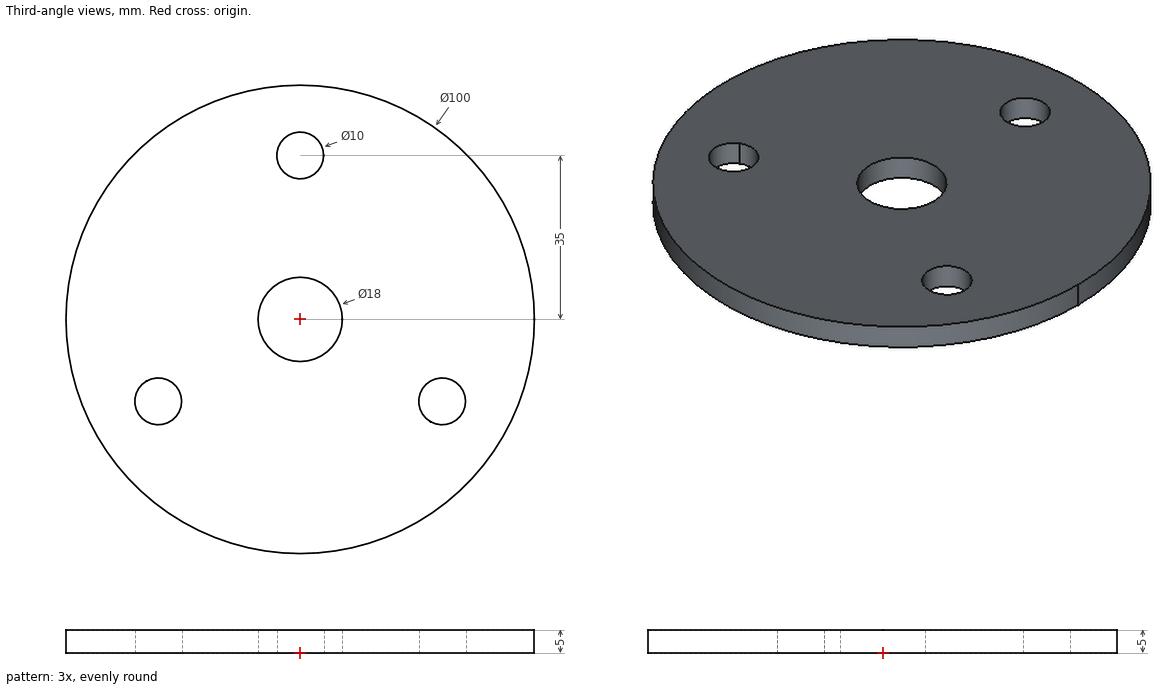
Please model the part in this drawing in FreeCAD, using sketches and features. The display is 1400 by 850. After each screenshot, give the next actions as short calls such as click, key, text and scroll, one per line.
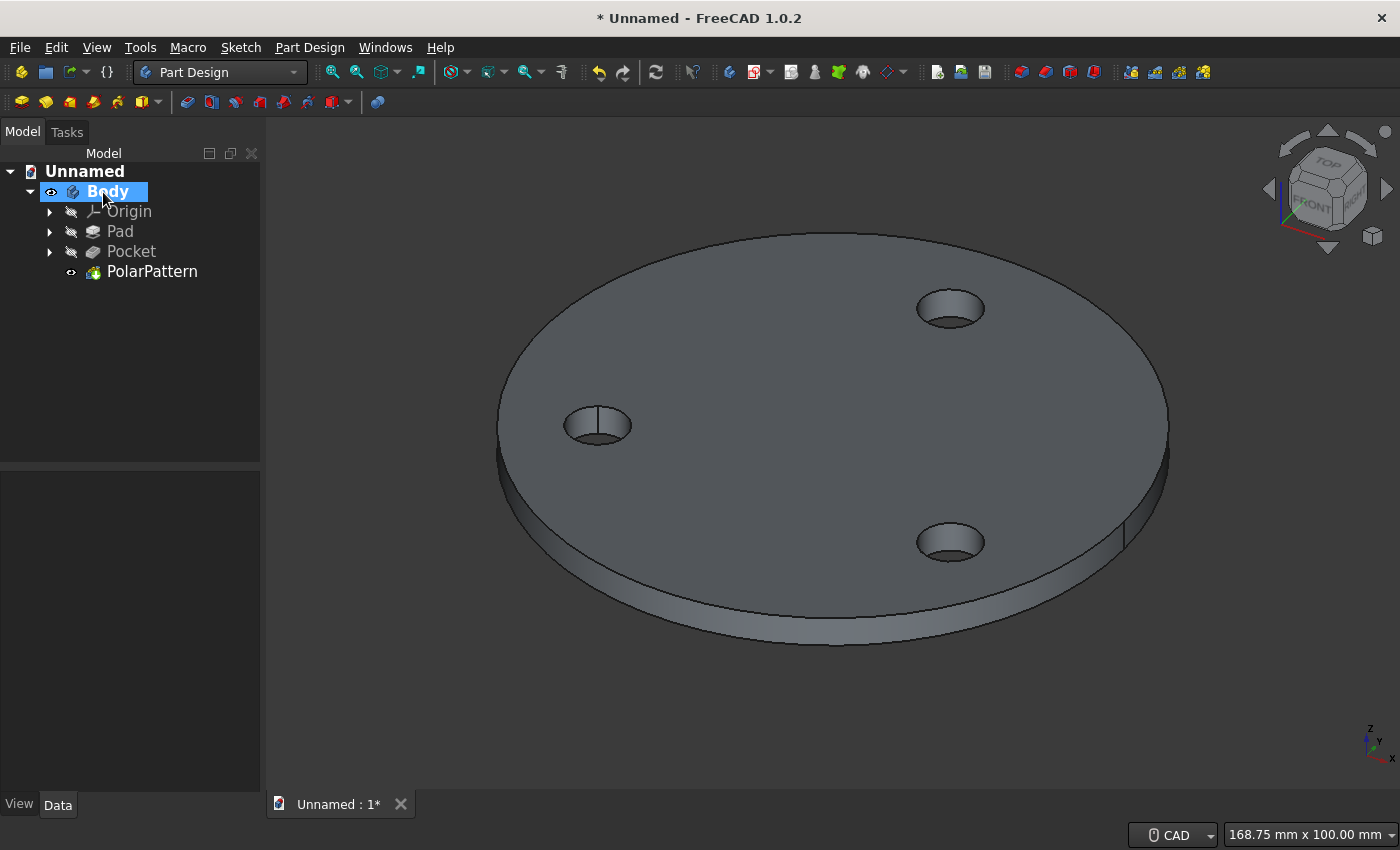
click(833, 424)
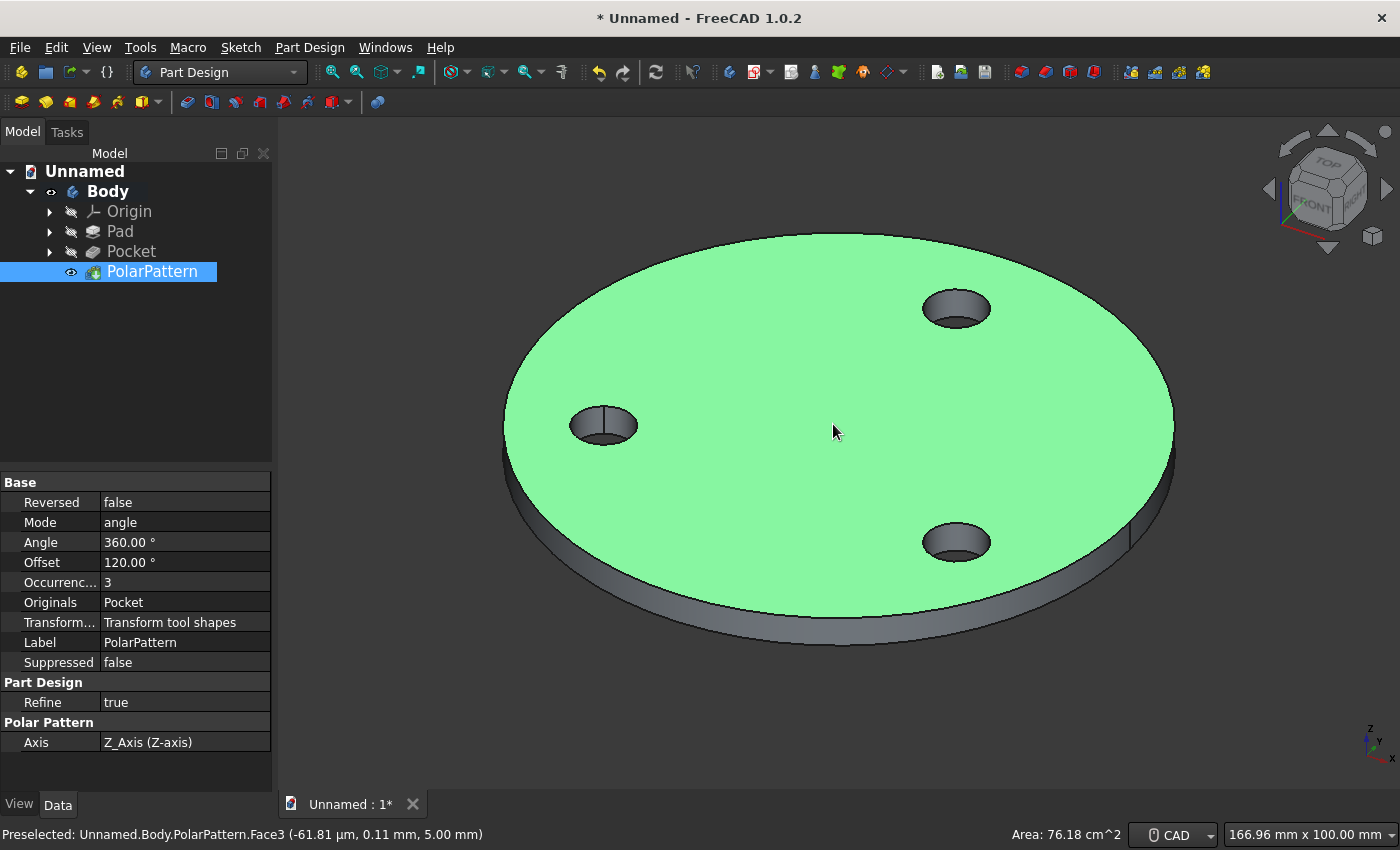
click(754, 72)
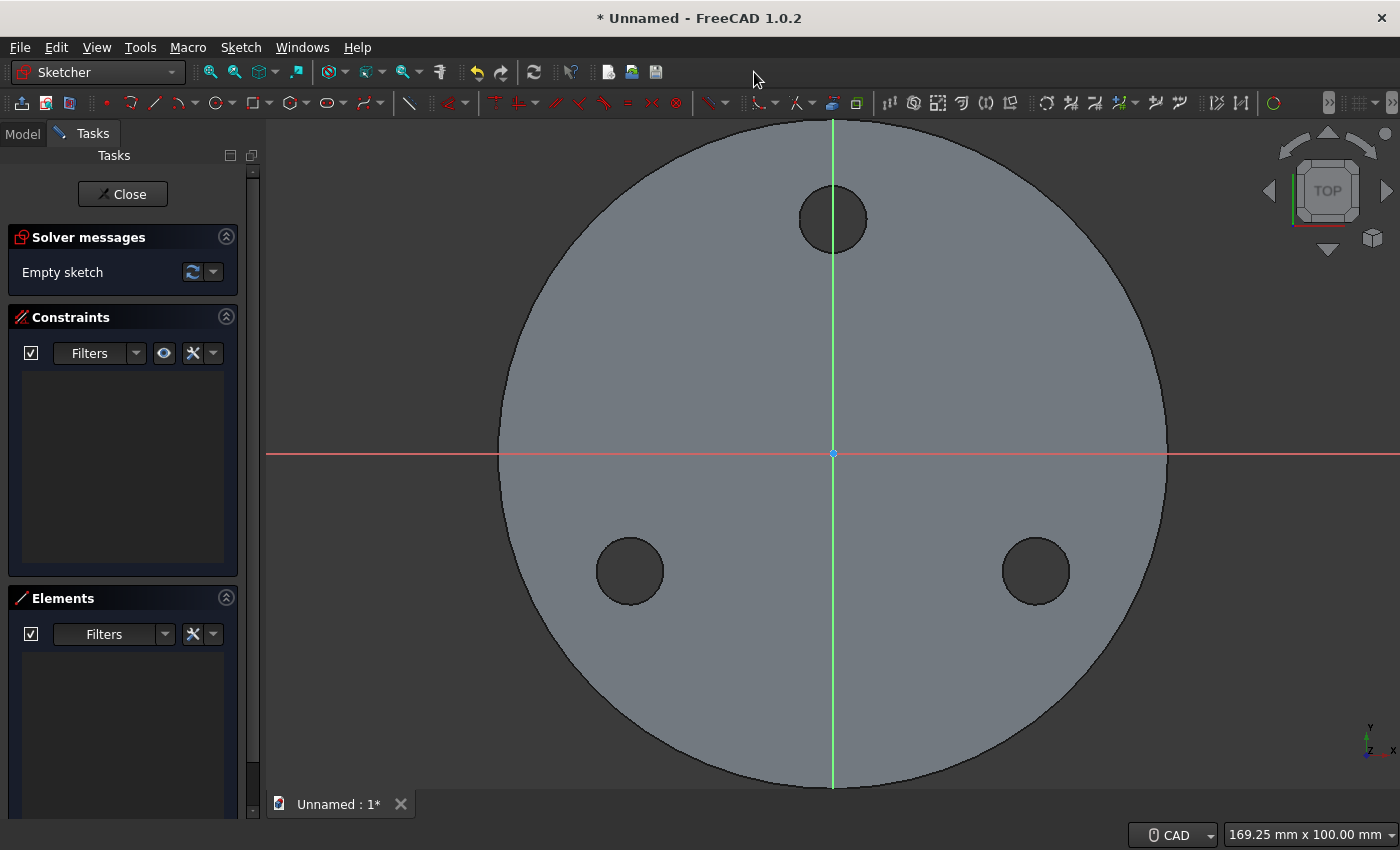
scroll(863, 454, up, 6)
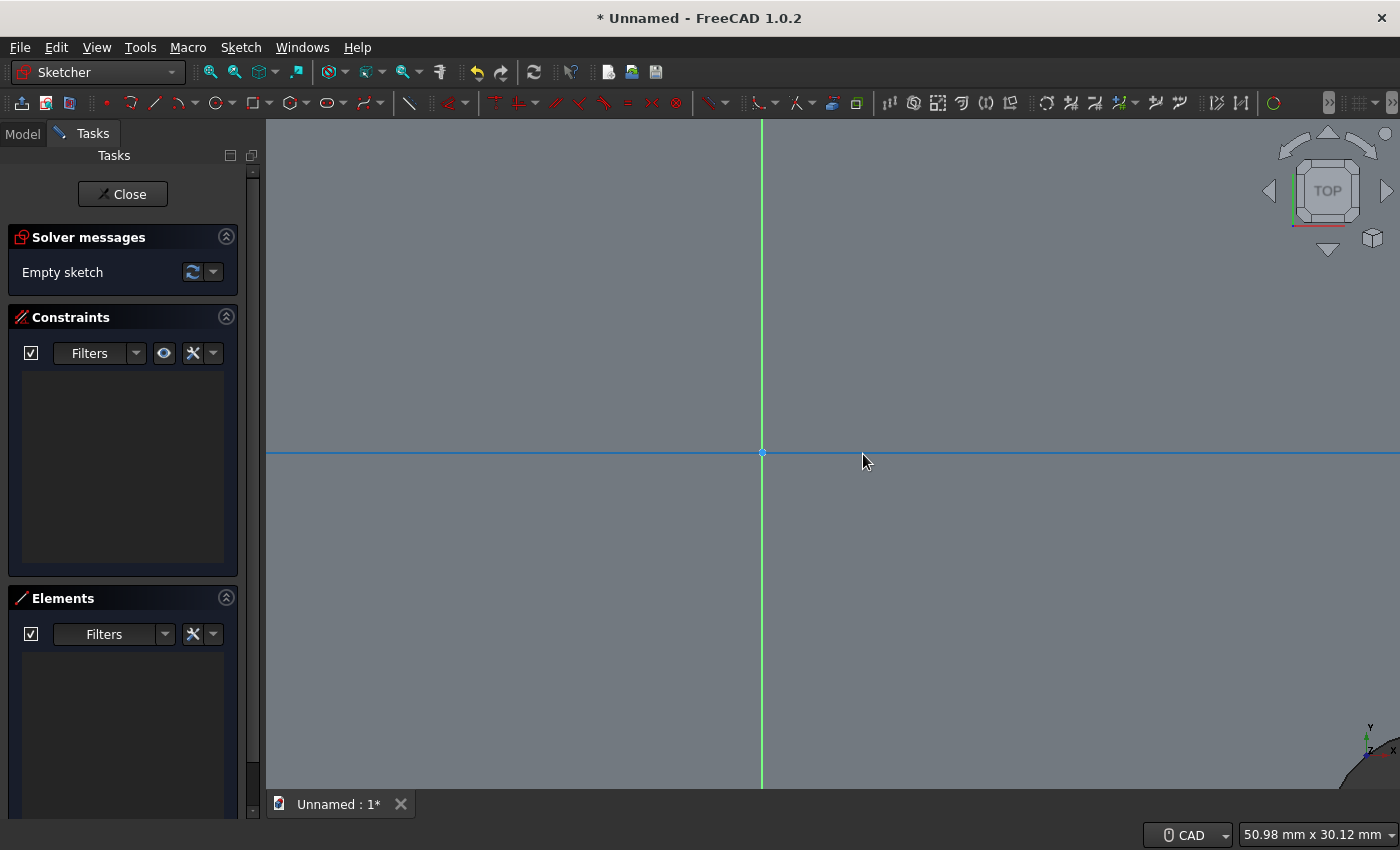
click(216, 104)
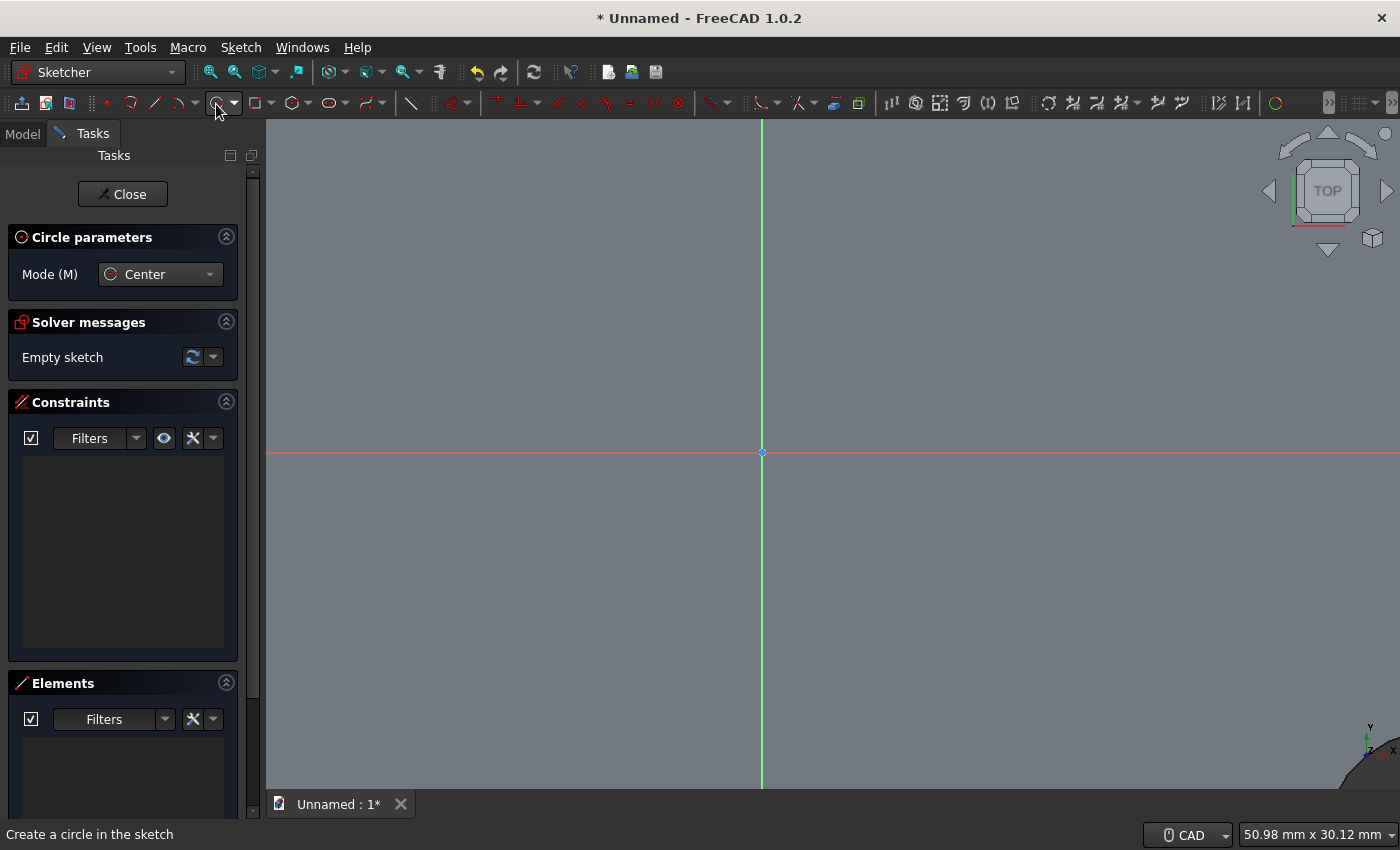
click(762, 453)
click(904, 311)
key(Escape)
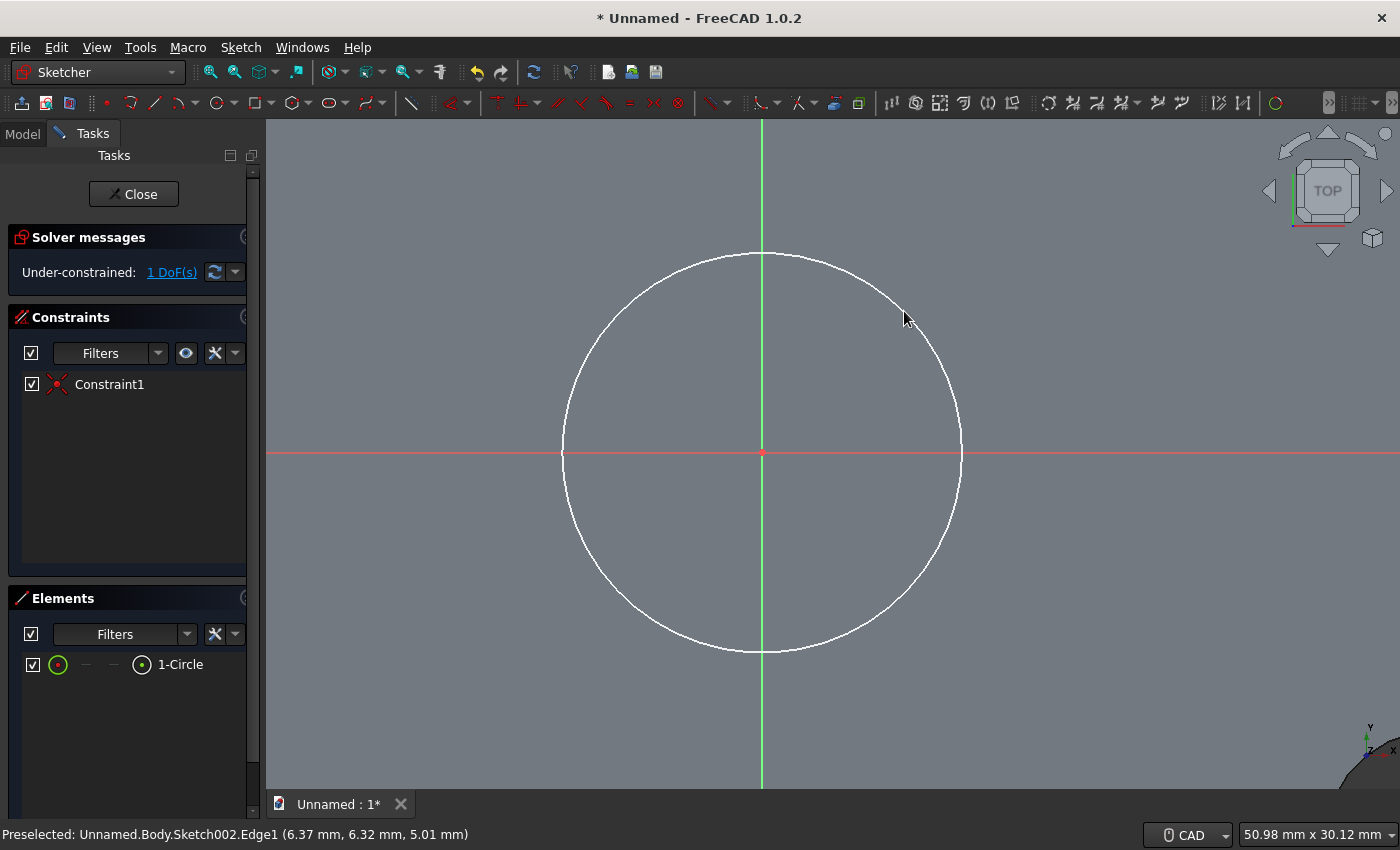
click(450, 104)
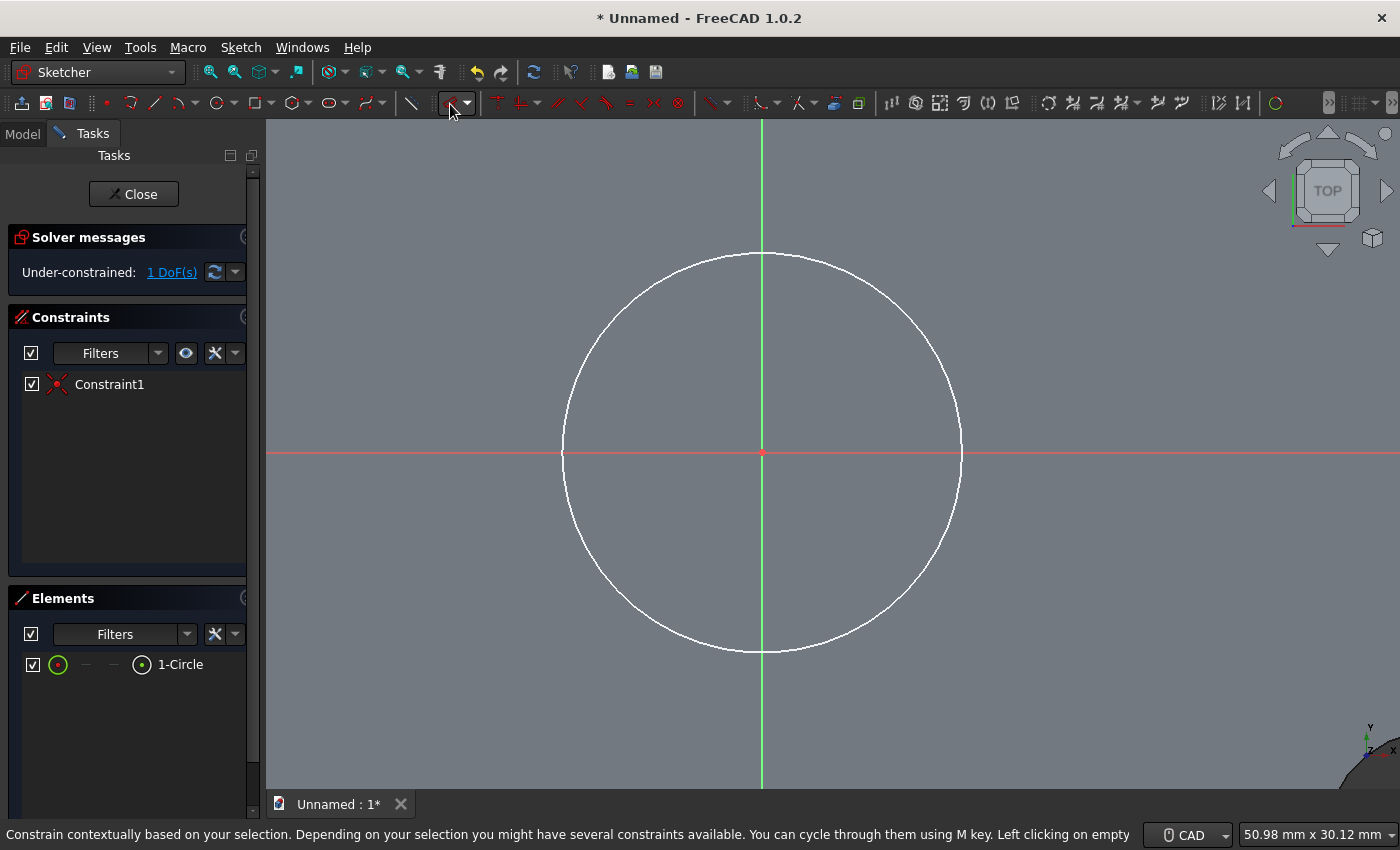
click(903, 311)
click(926, 288)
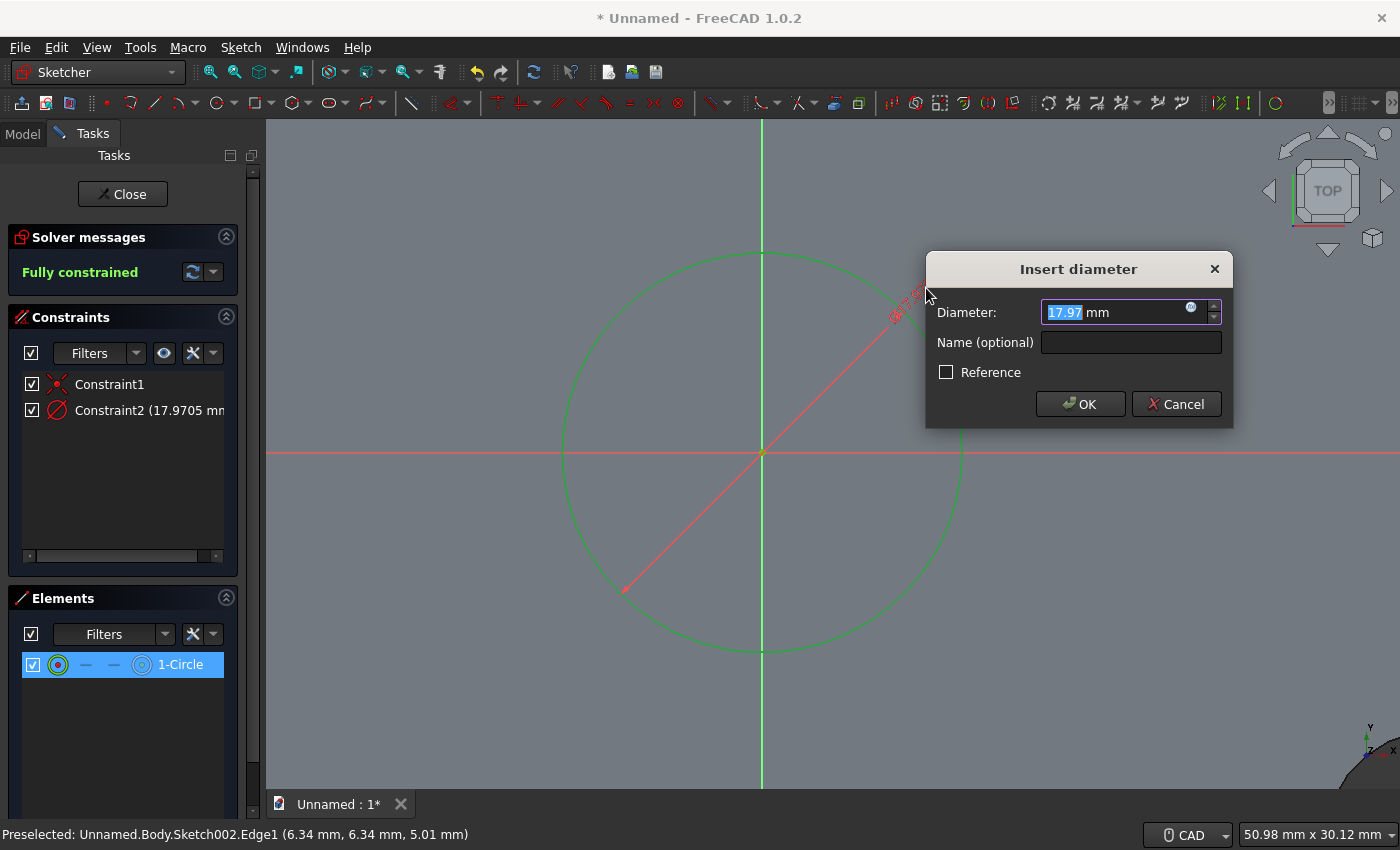
text(18)
key(Return)
key(Escape)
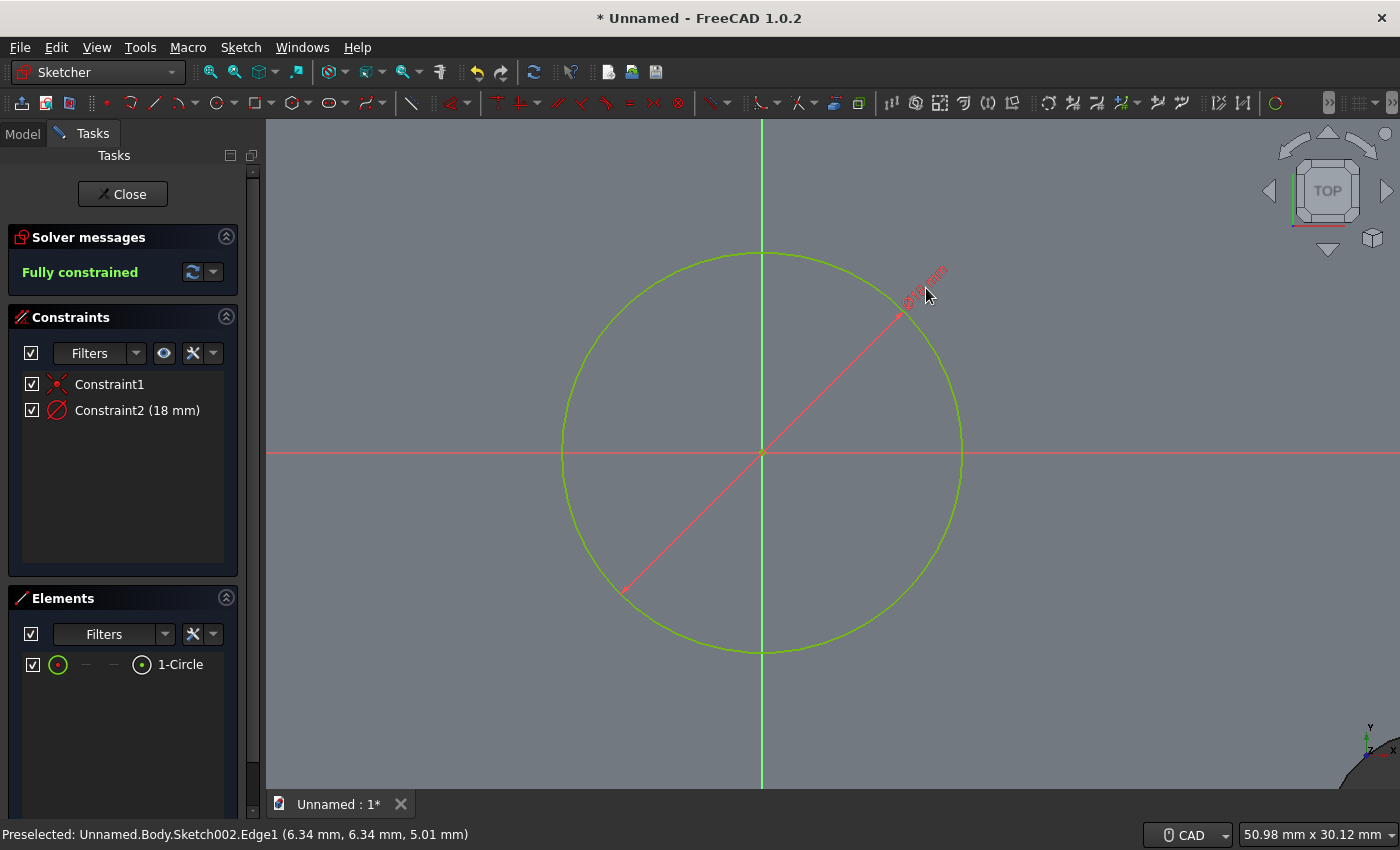
click(123, 194)